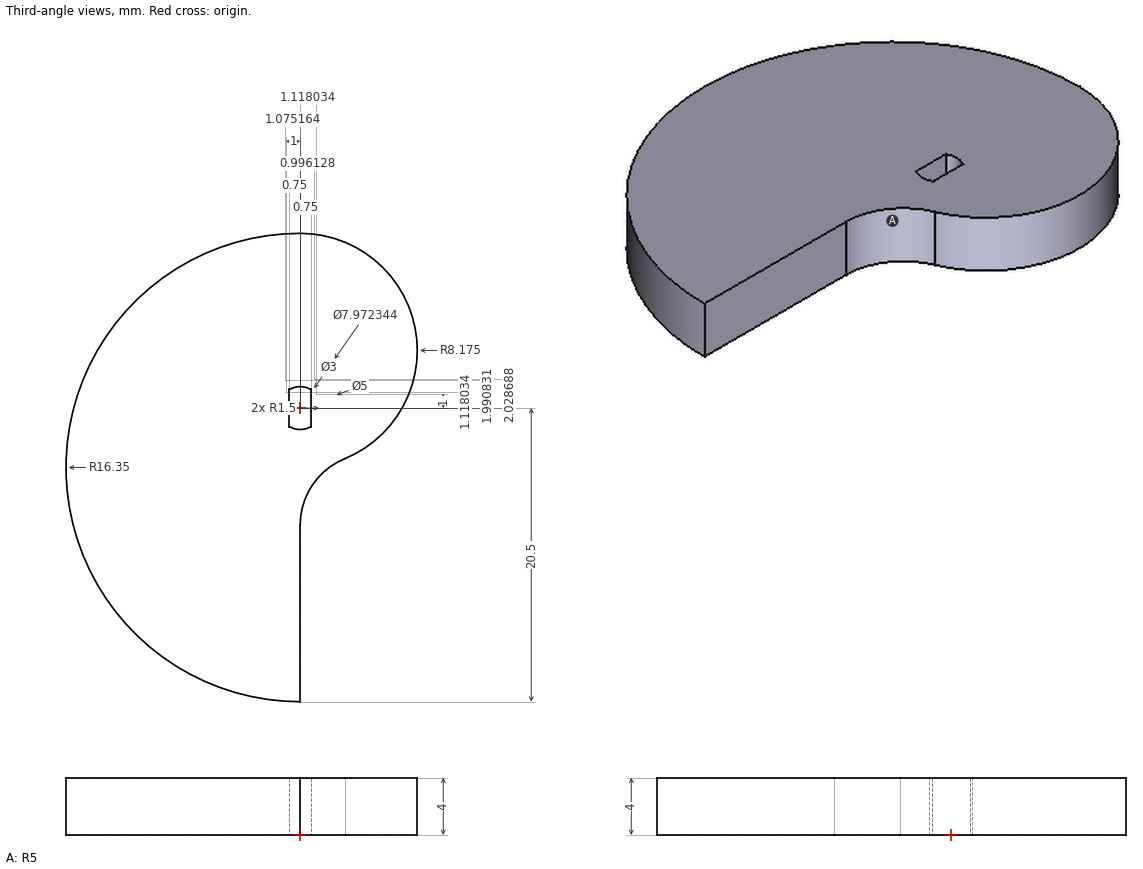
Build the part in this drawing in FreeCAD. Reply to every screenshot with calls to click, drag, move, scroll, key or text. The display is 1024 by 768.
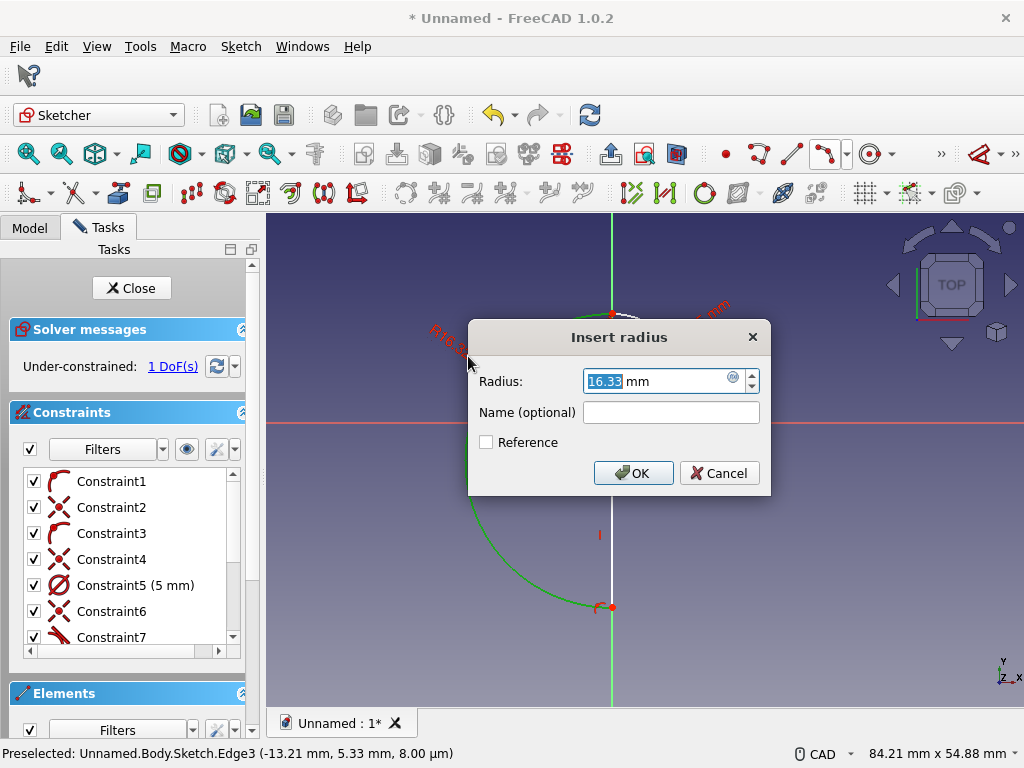
text(16.35)
key(Return)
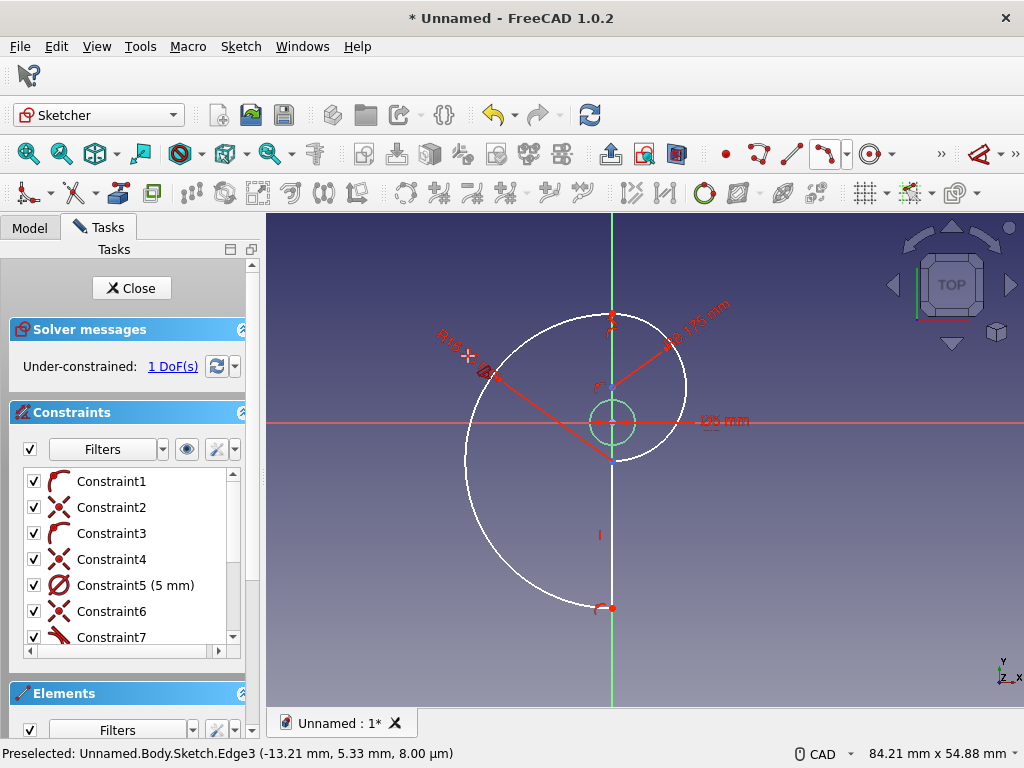
click(612, 608)
click(646, 515)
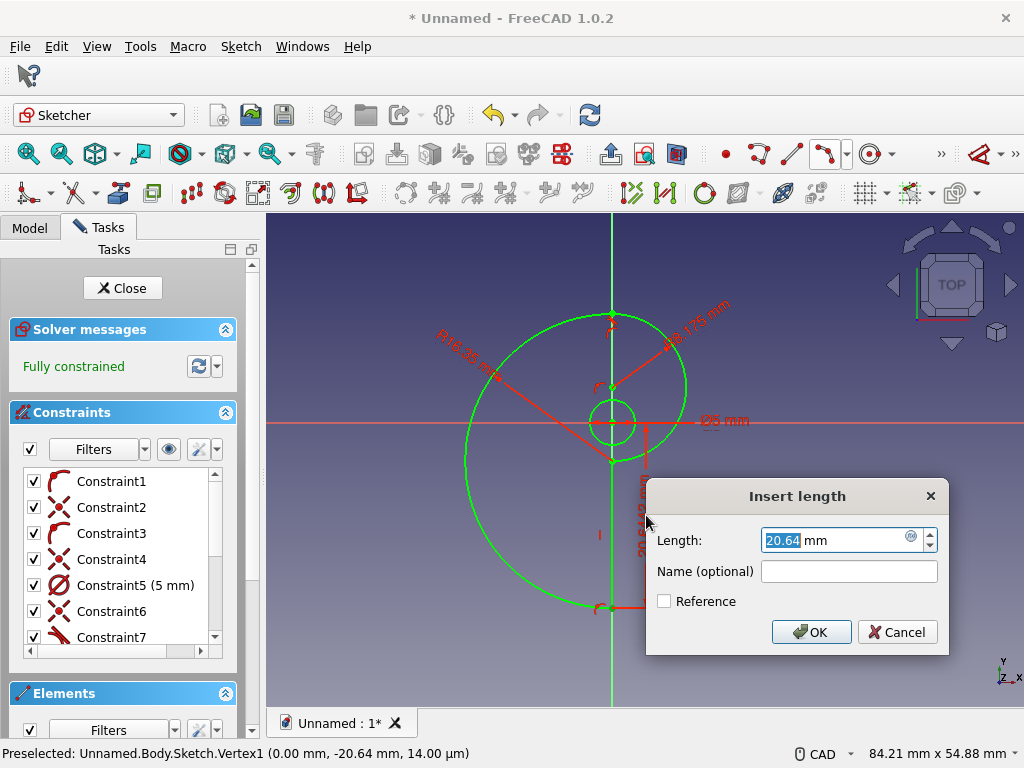
text(20.5)
key(Return)
key(Escape)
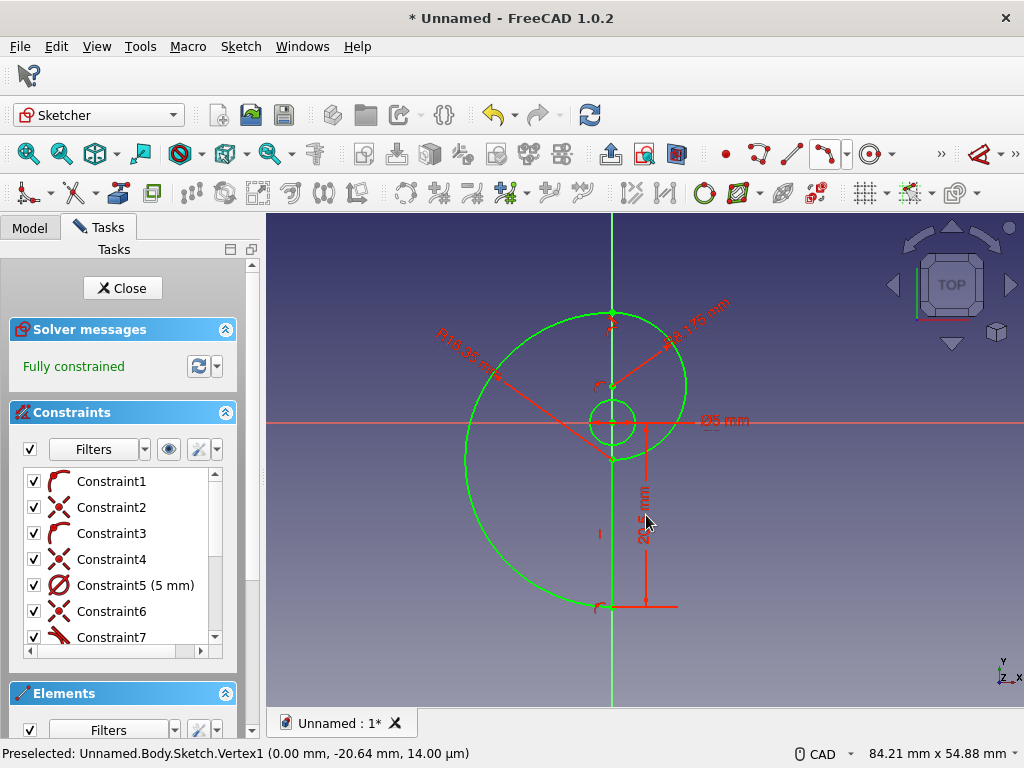
click(123, 288)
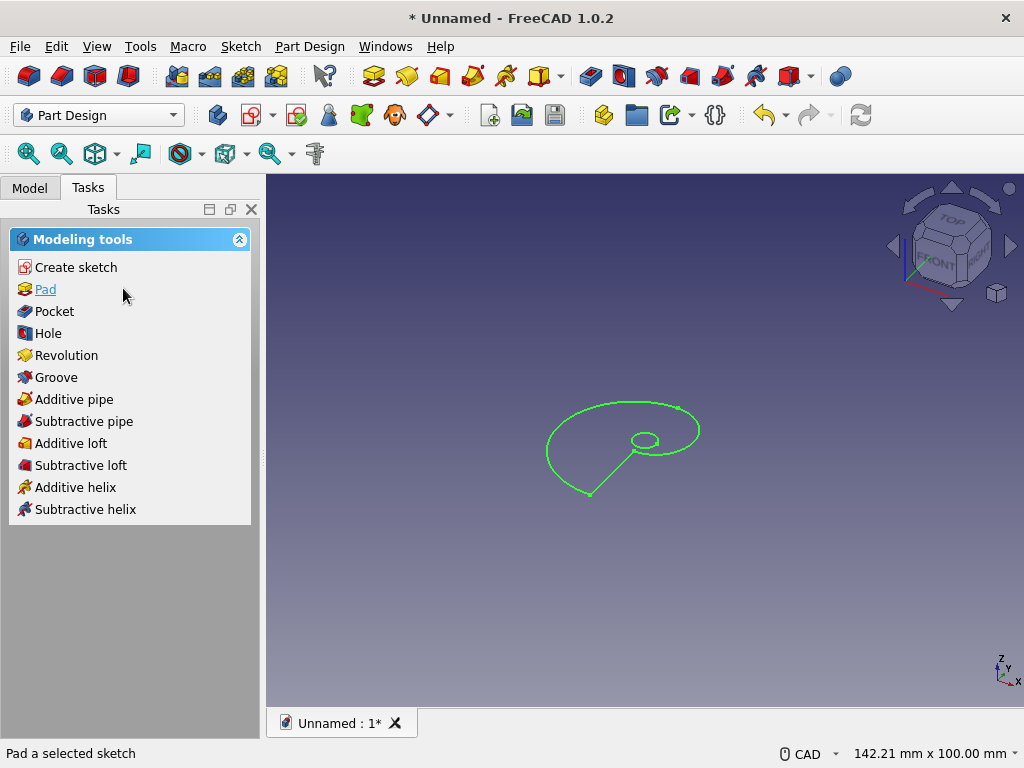
click(374, 76)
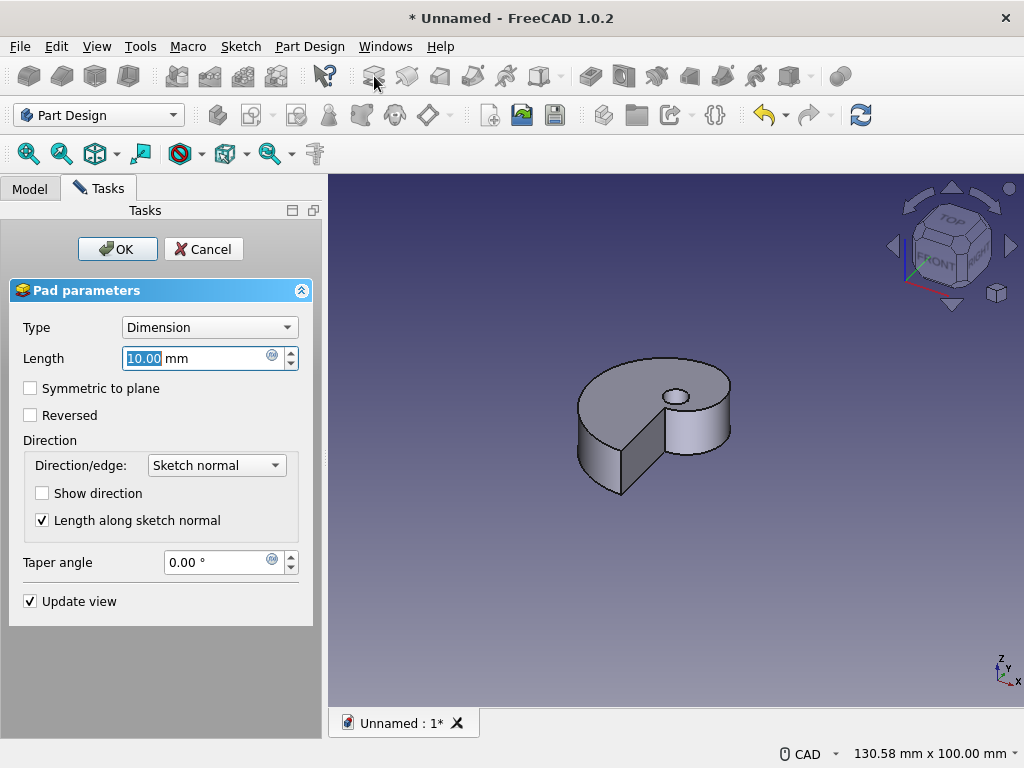
text(4)
key(Tab)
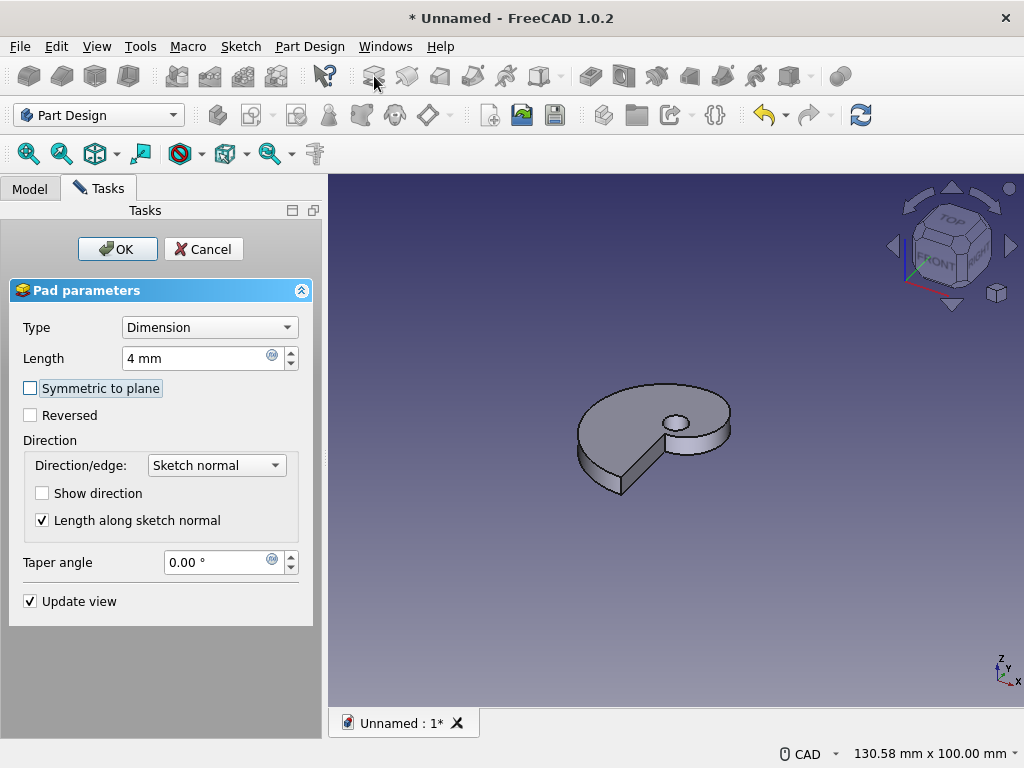
click(118, 249)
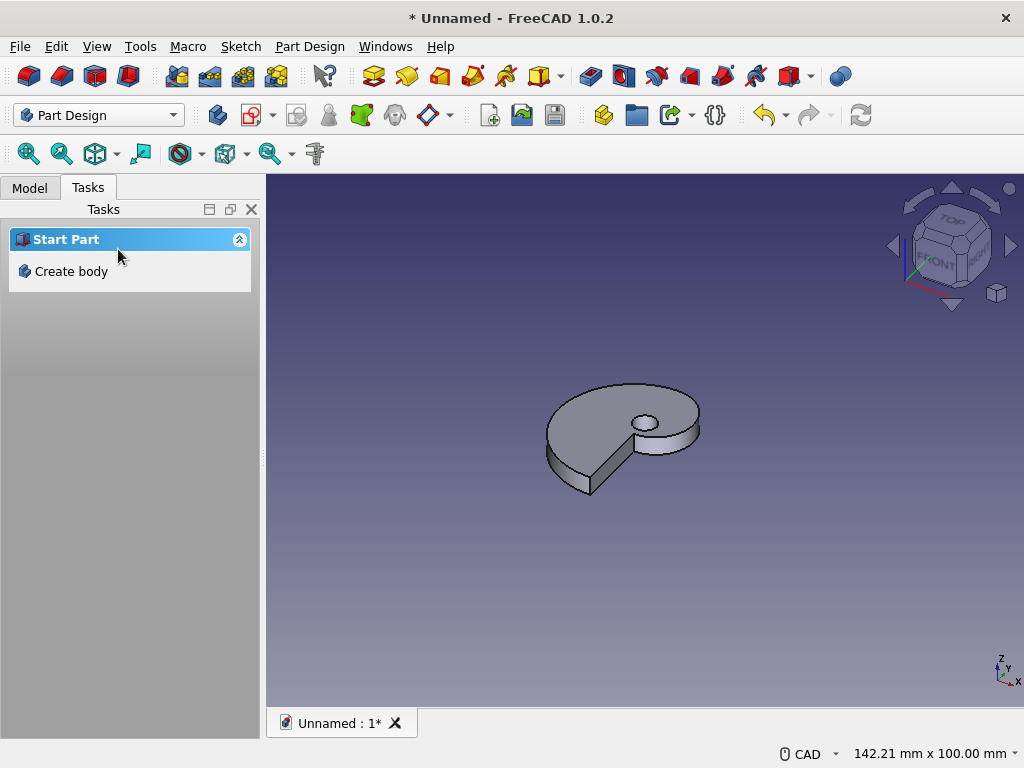
key(v)
key(f)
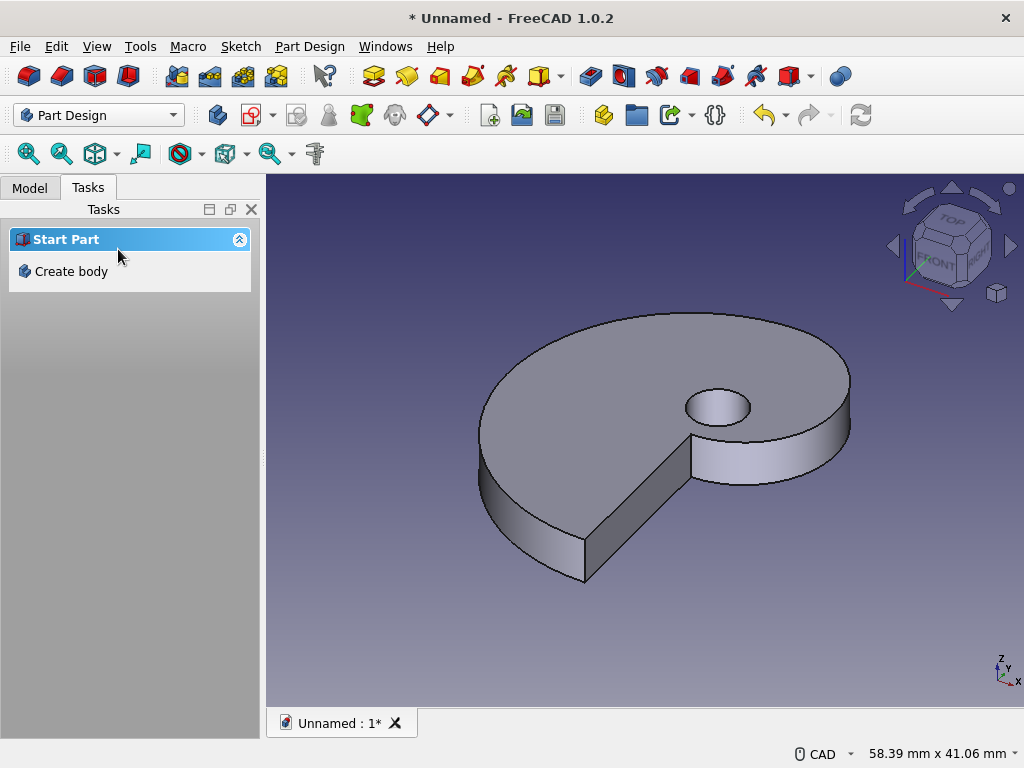
key(0)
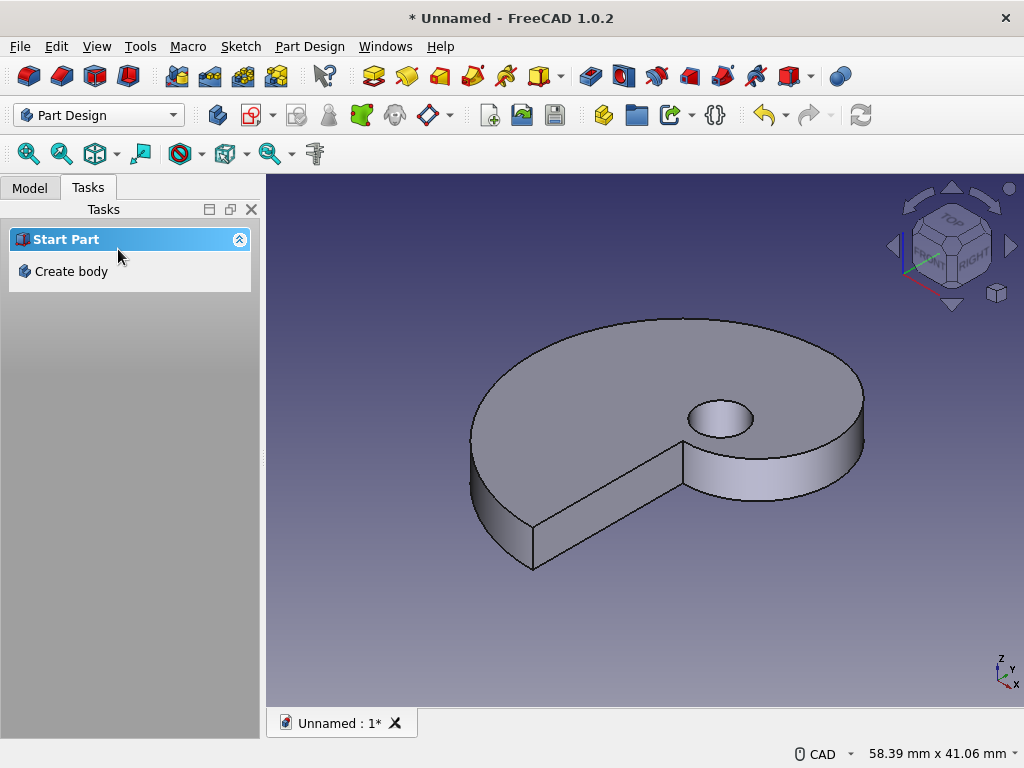
key(2)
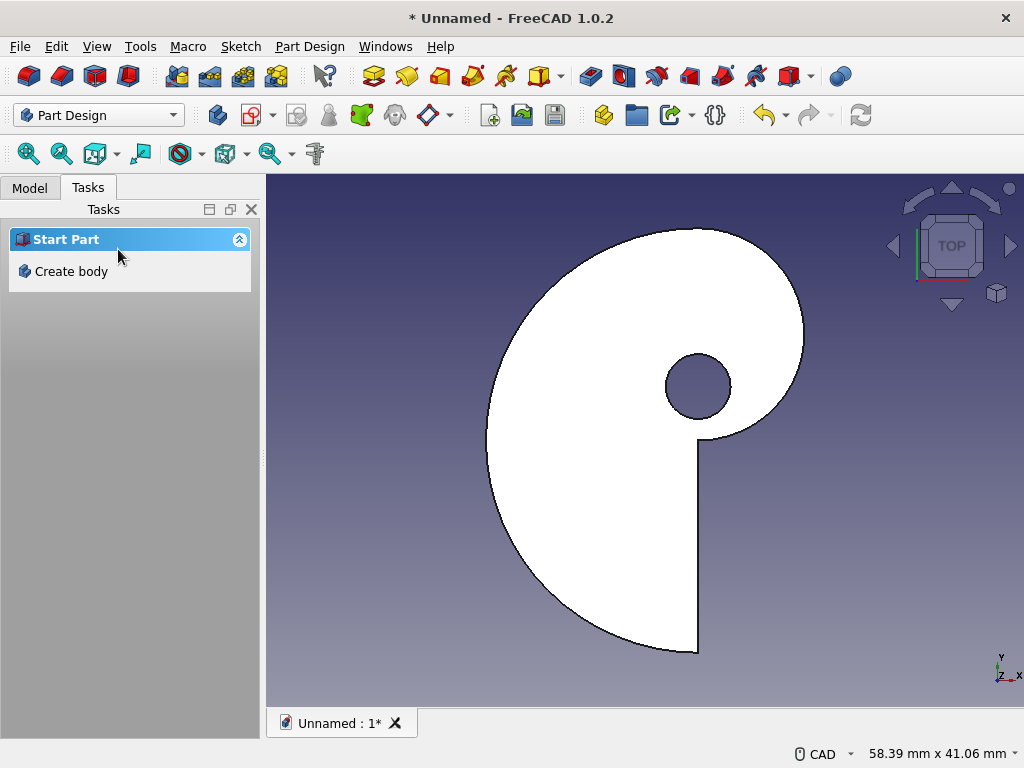
key(1)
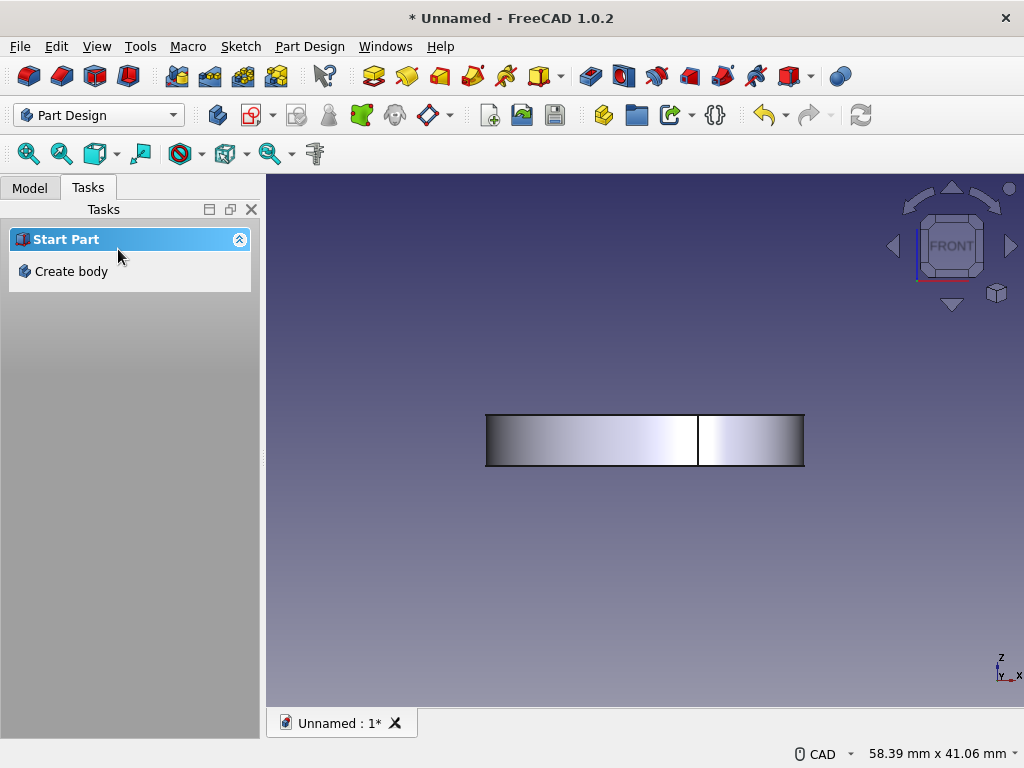
key(v)
key(f)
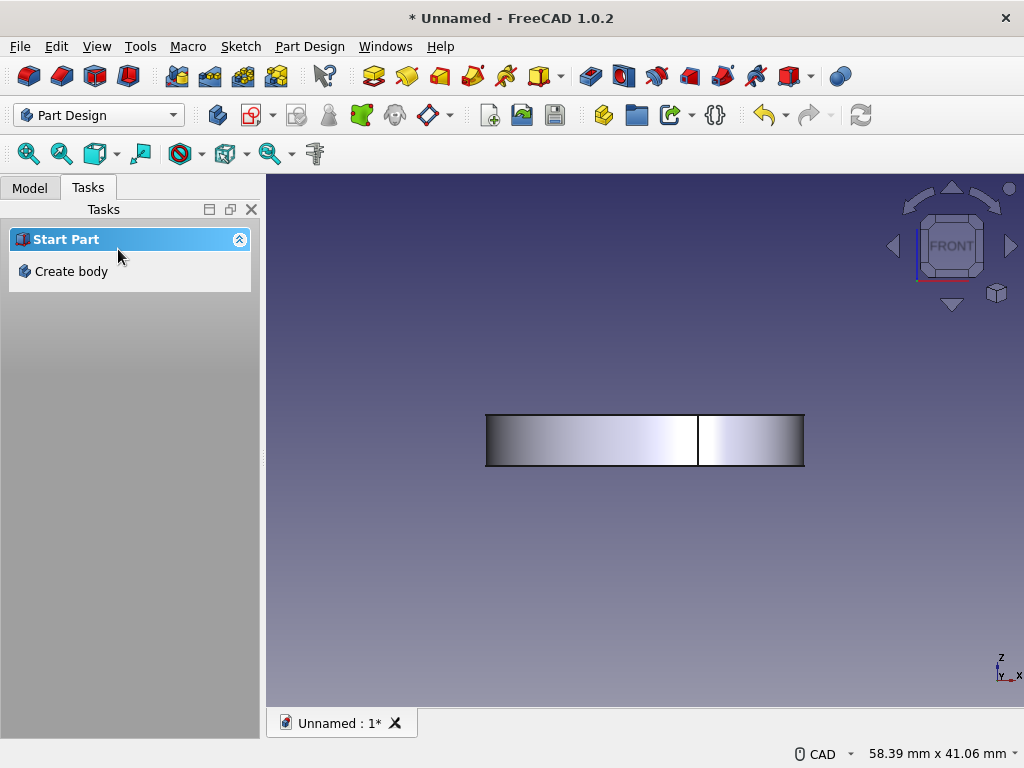
key(3)